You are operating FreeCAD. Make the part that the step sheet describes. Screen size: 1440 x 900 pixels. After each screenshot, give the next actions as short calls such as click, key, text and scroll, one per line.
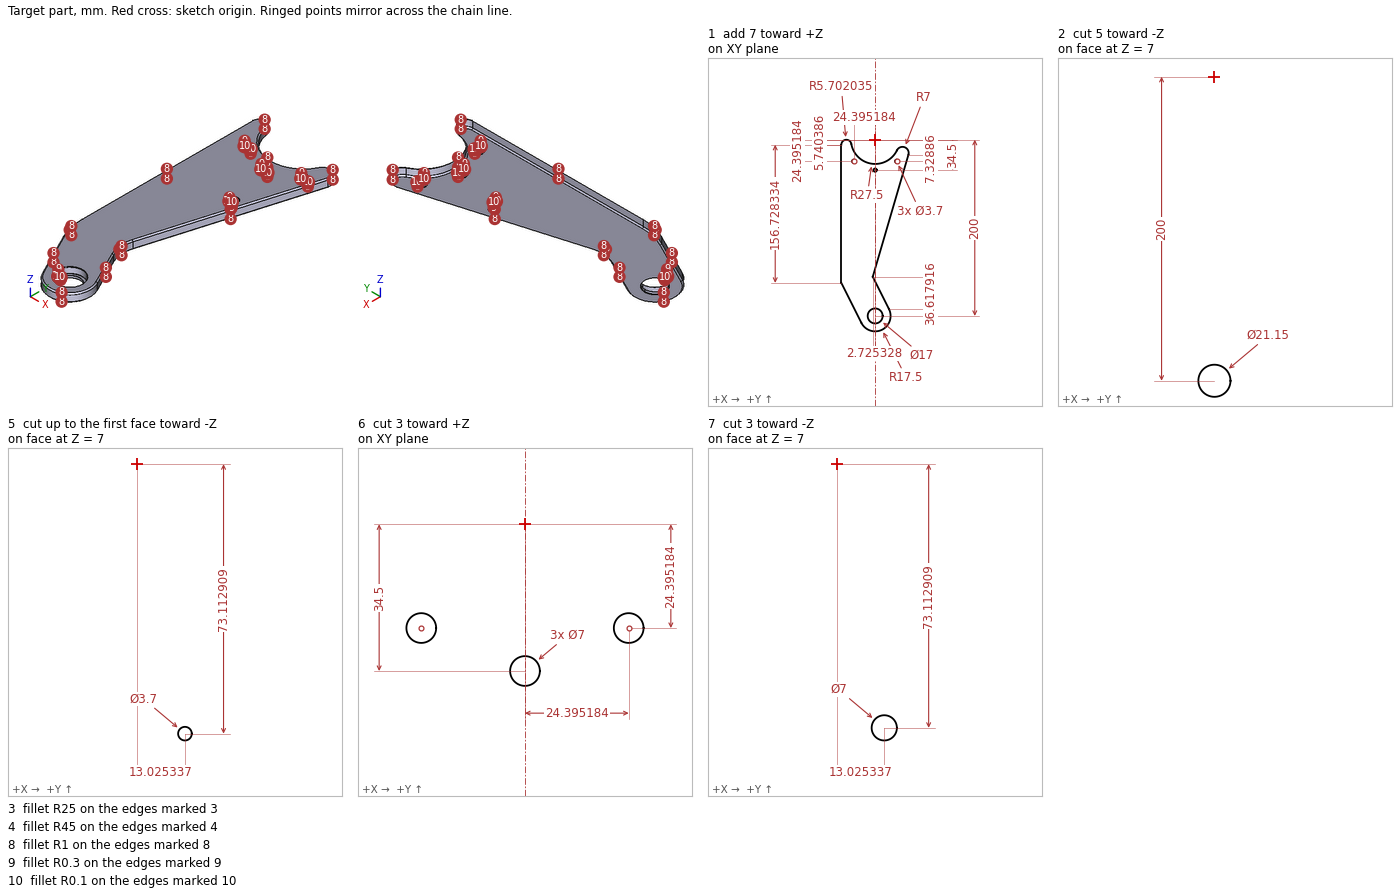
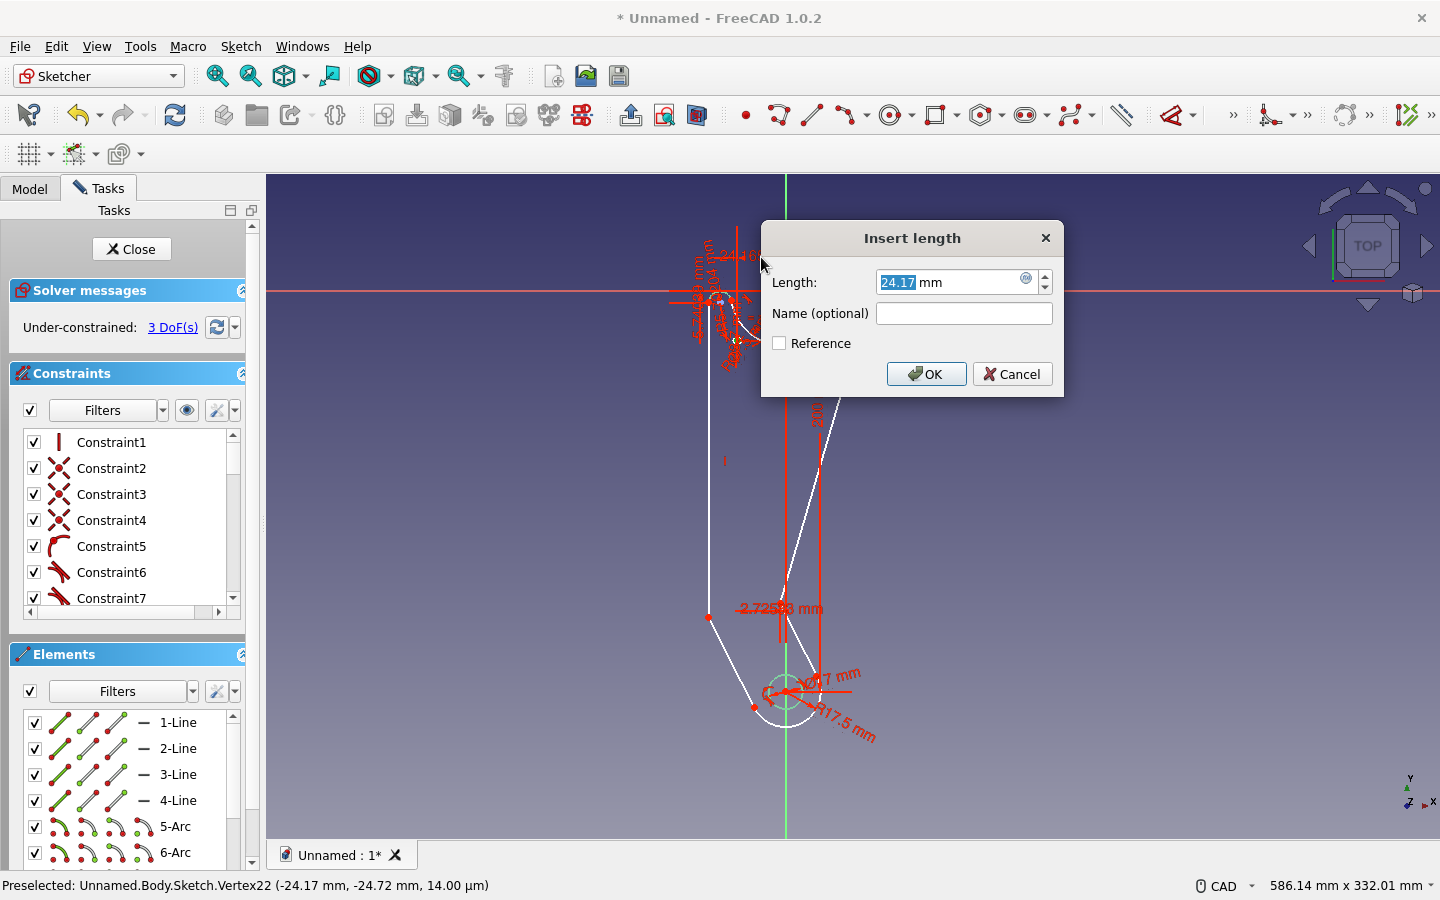
text(24.395184)
key(Return)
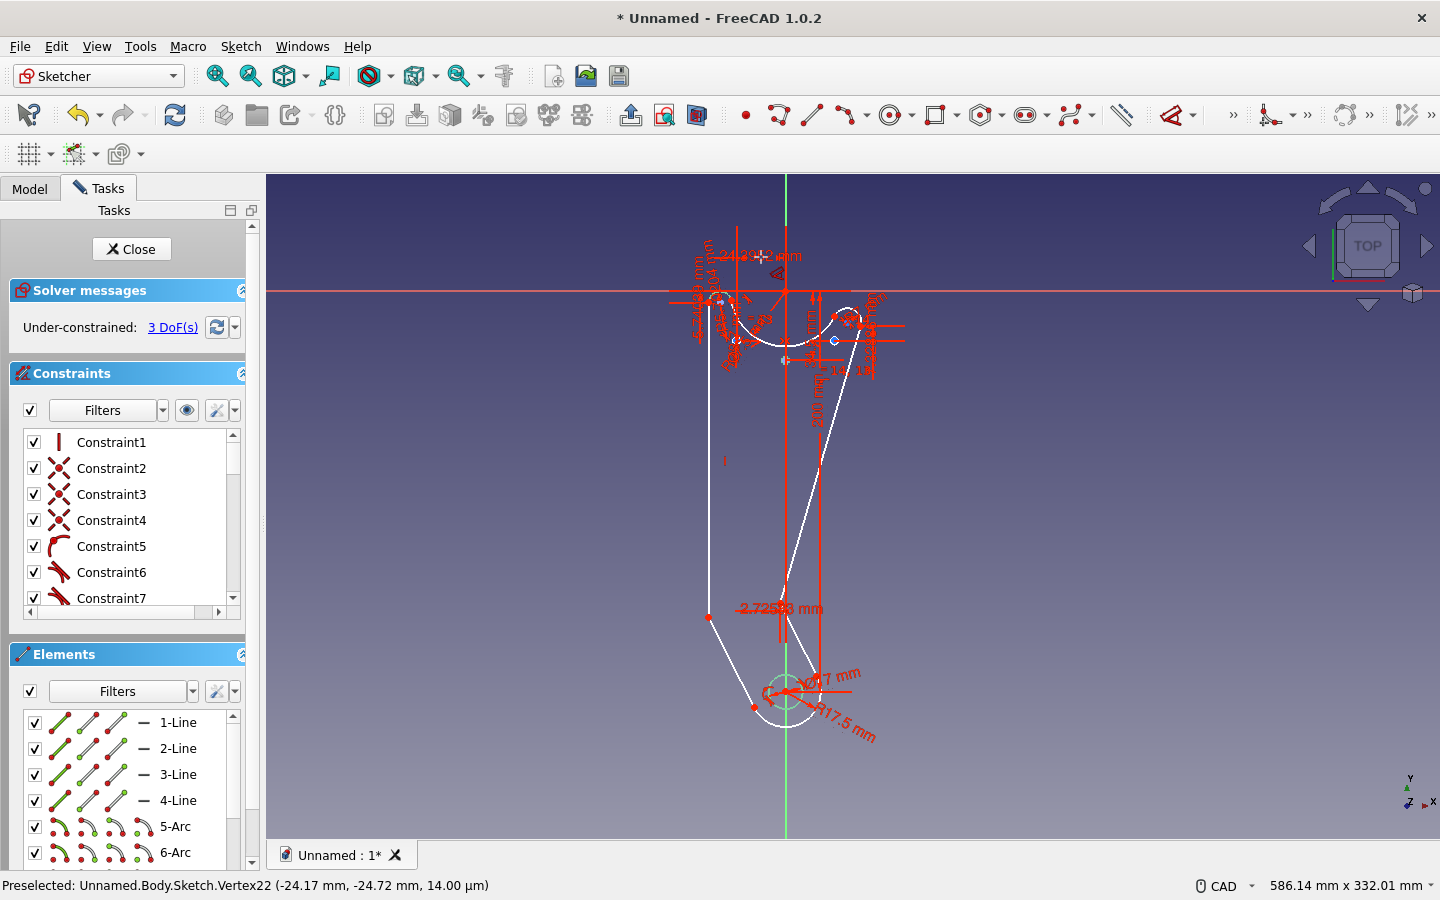
click(737, 341)
click(655, 328)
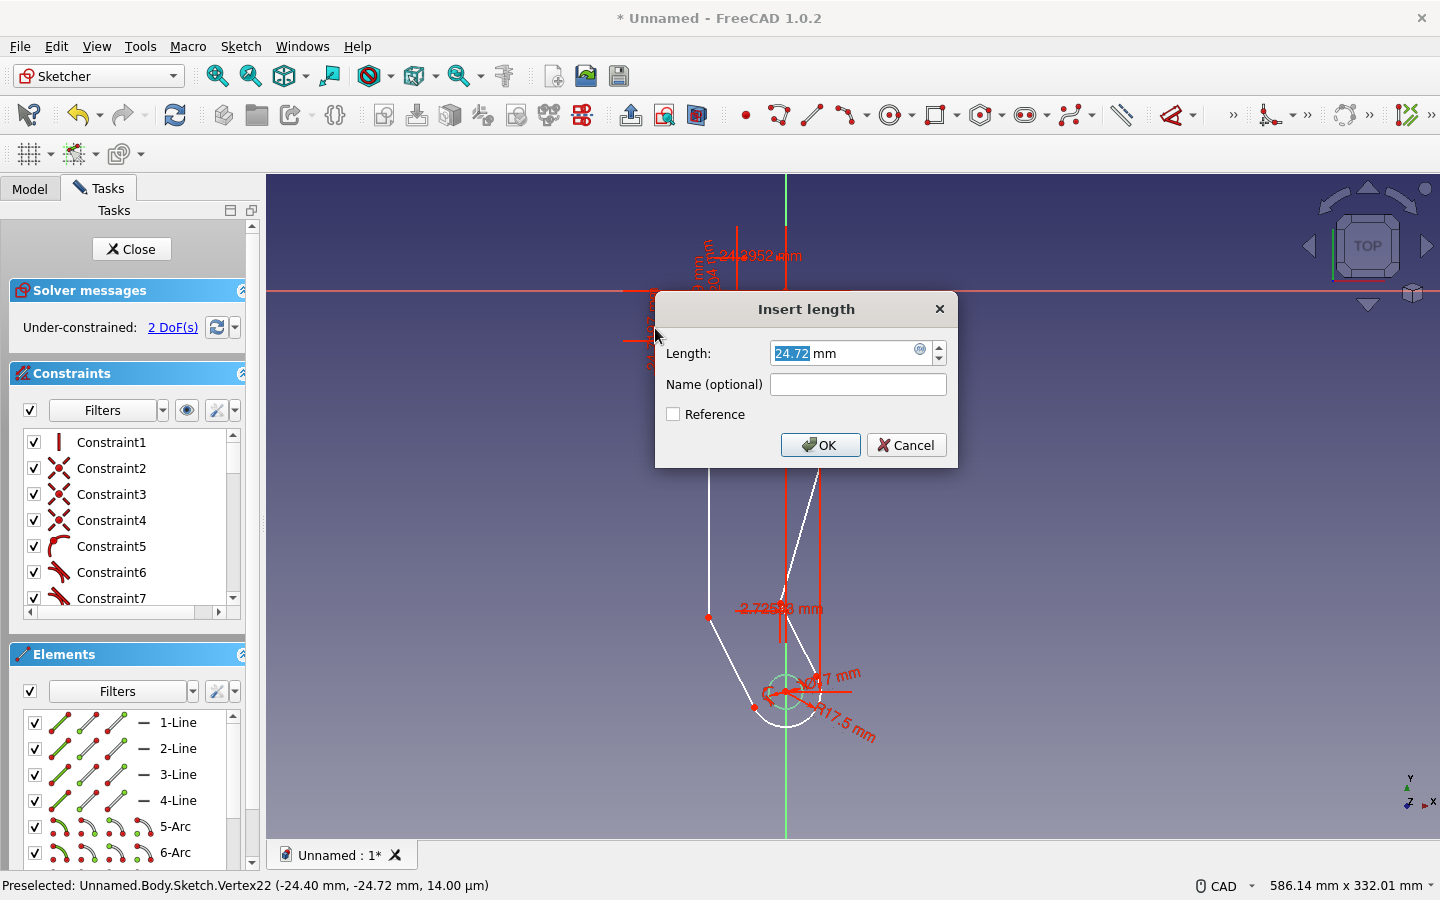
text(24.395184)
key(Return)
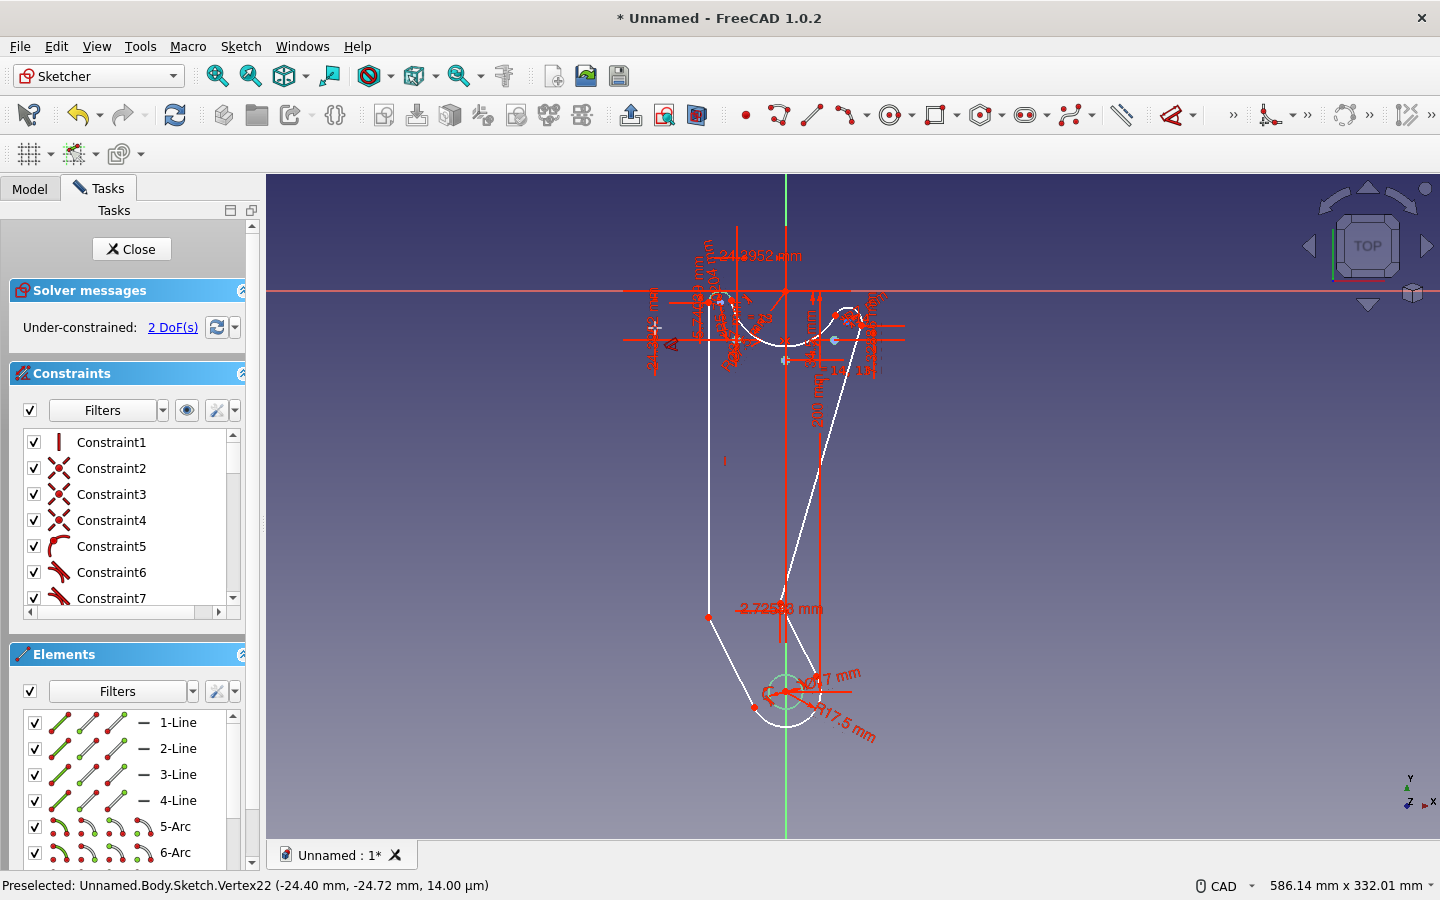
click(709, 397)
click(675, 460)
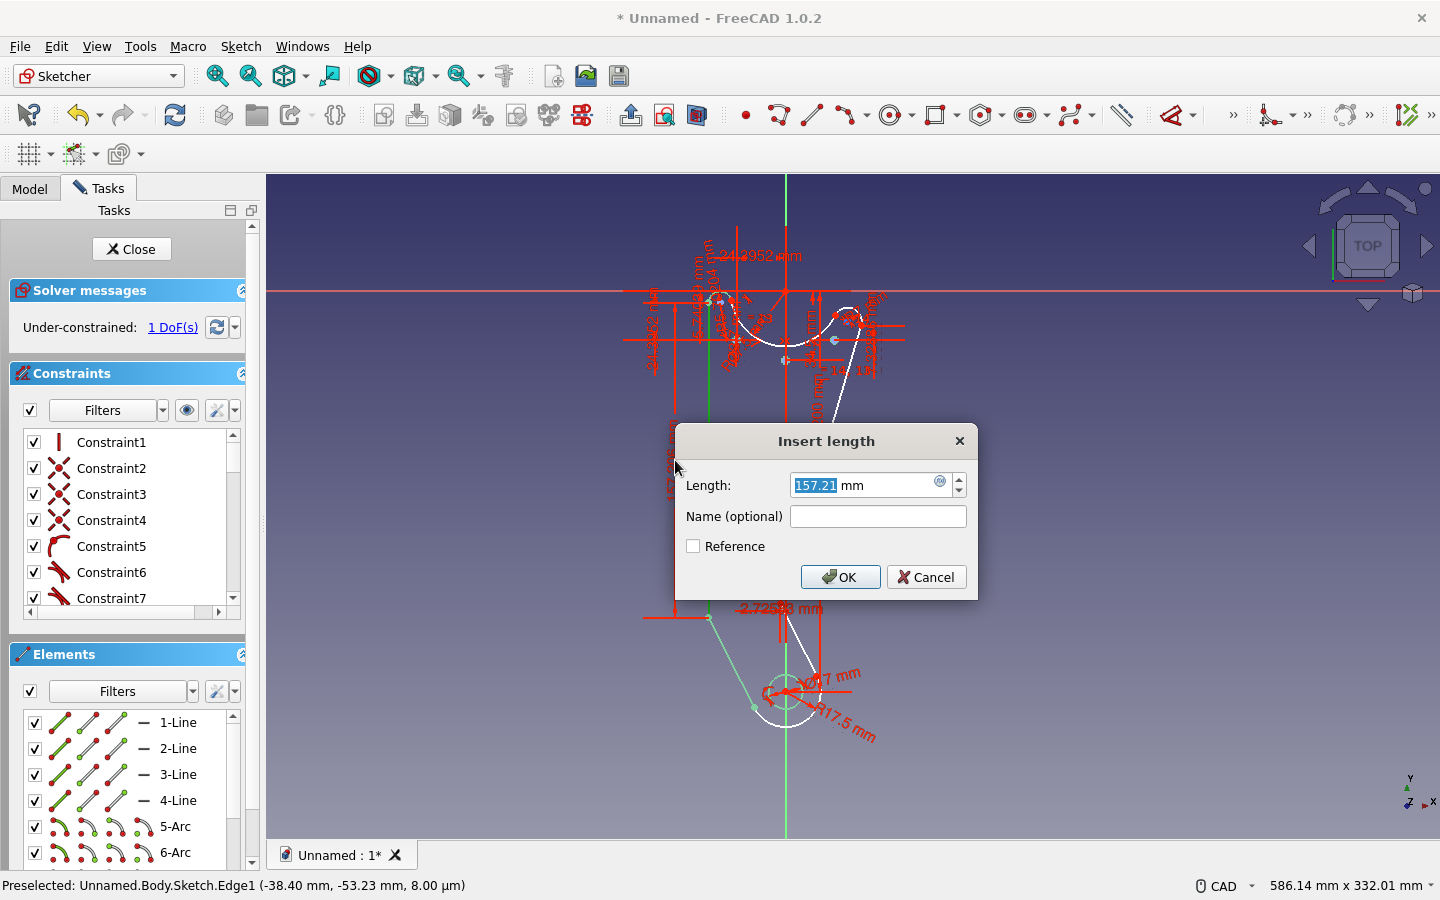
text(156.728334)
key(Return)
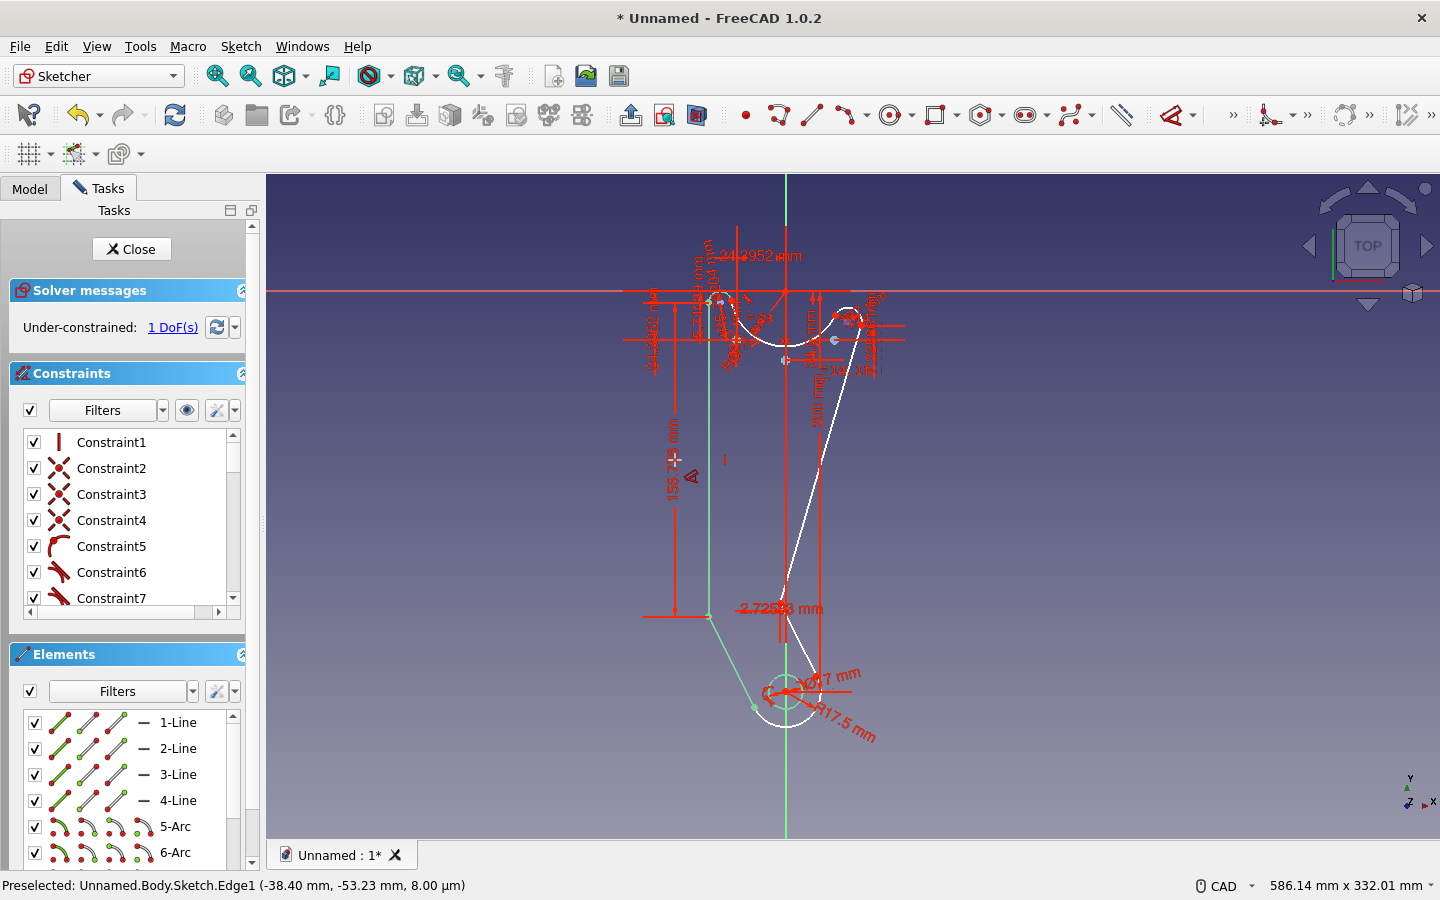
click(806, 654)
click(851, 640)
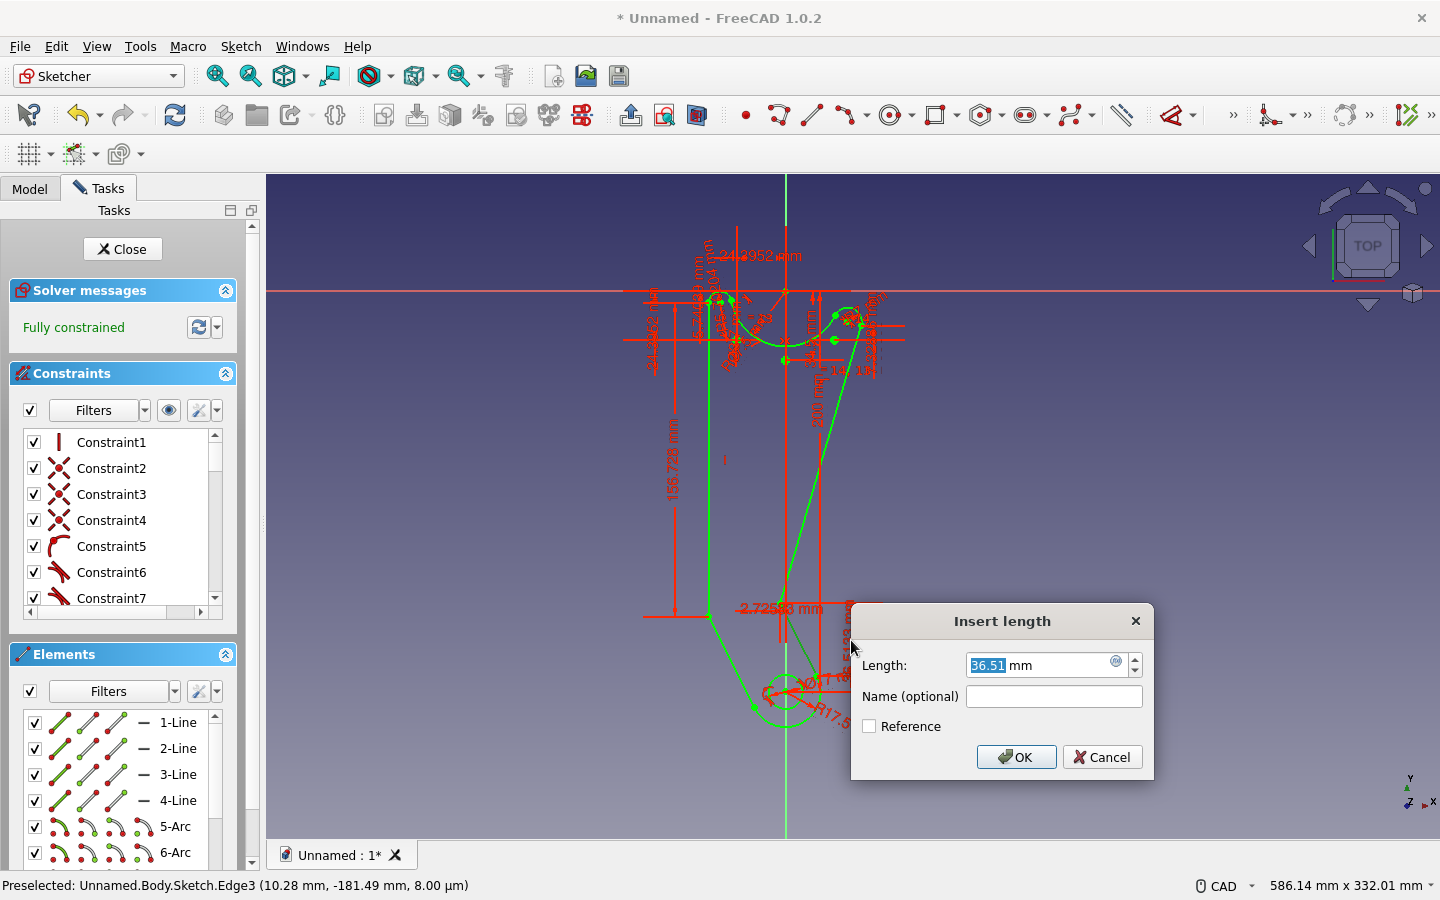
text(36.617916)
key(Return)
key(Escape)